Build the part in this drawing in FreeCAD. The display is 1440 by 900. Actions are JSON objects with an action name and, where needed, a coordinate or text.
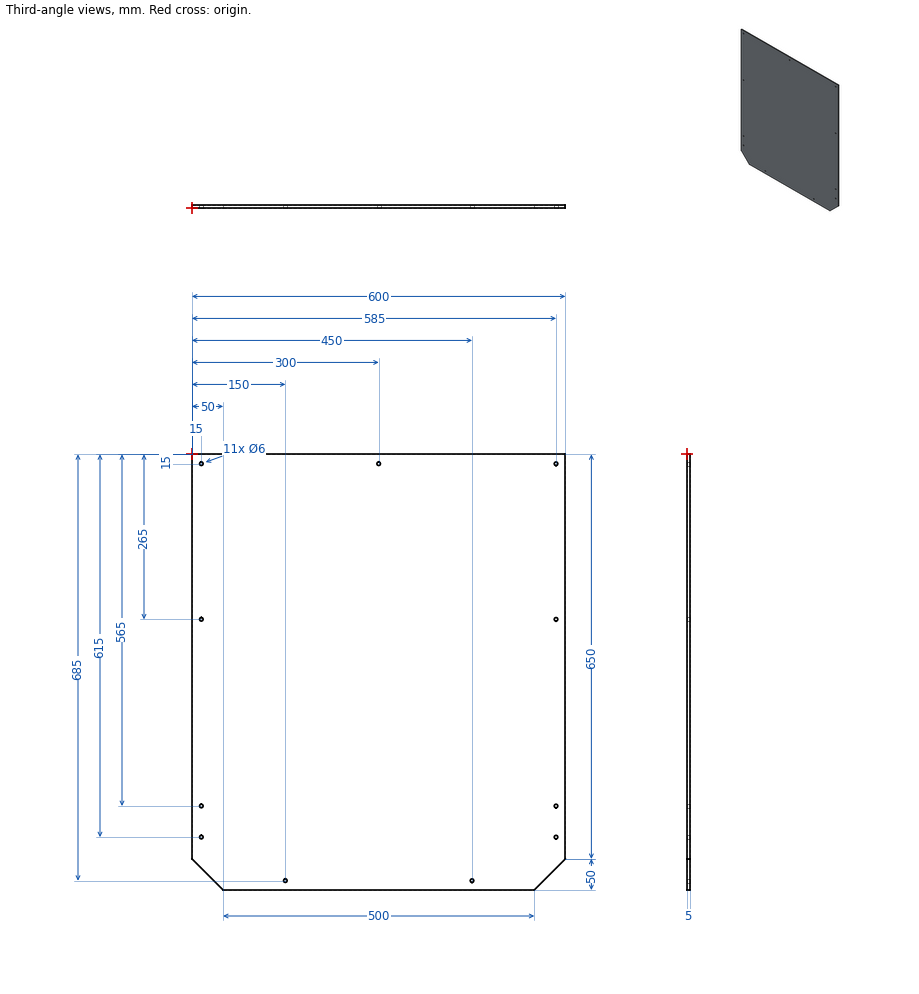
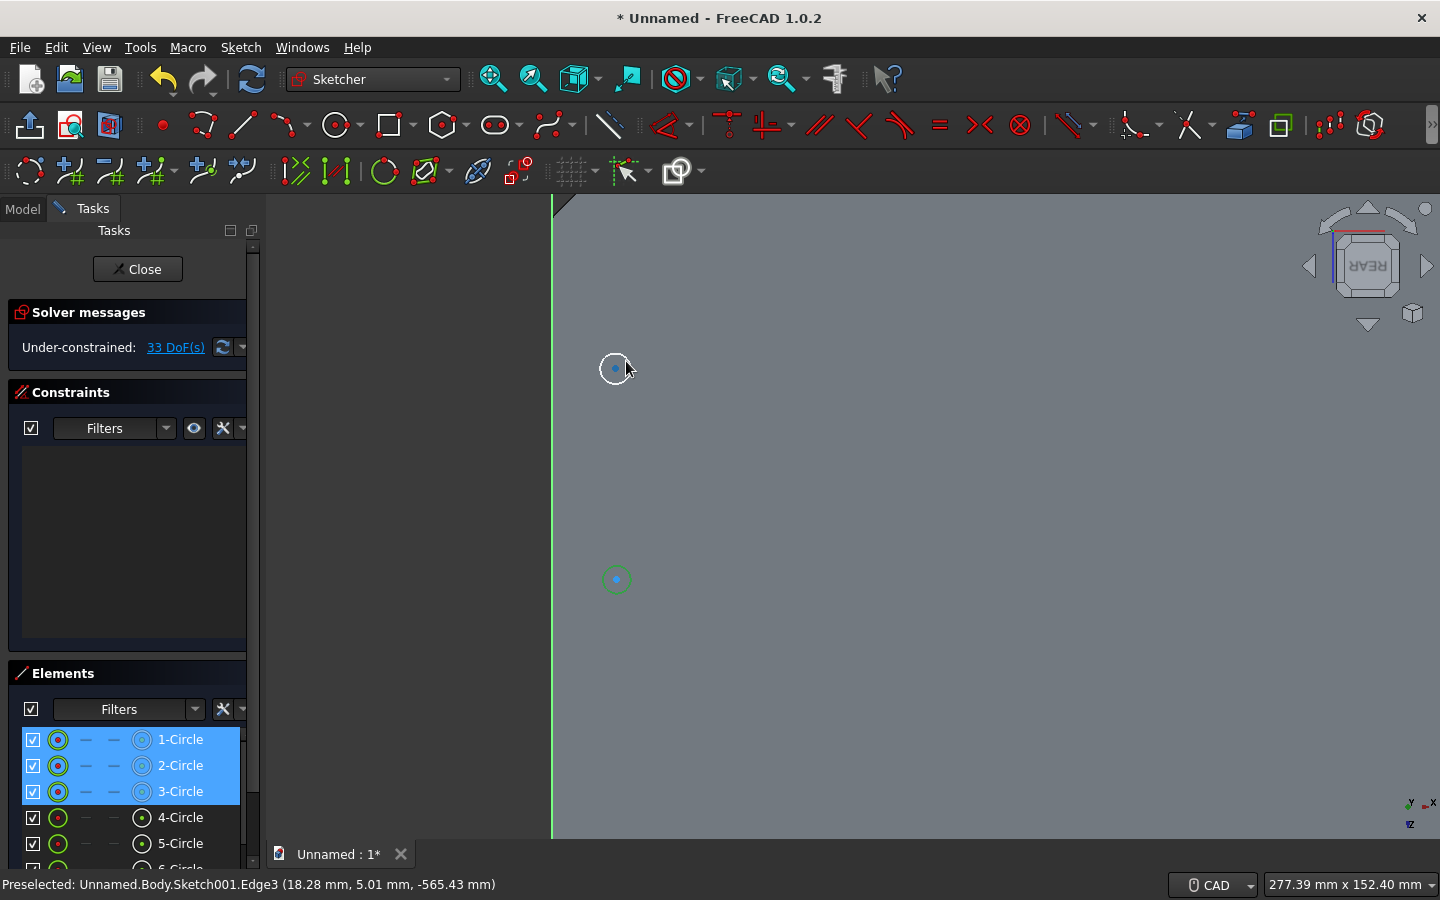
{"action": "left_click", "coordinate": [626, 358]}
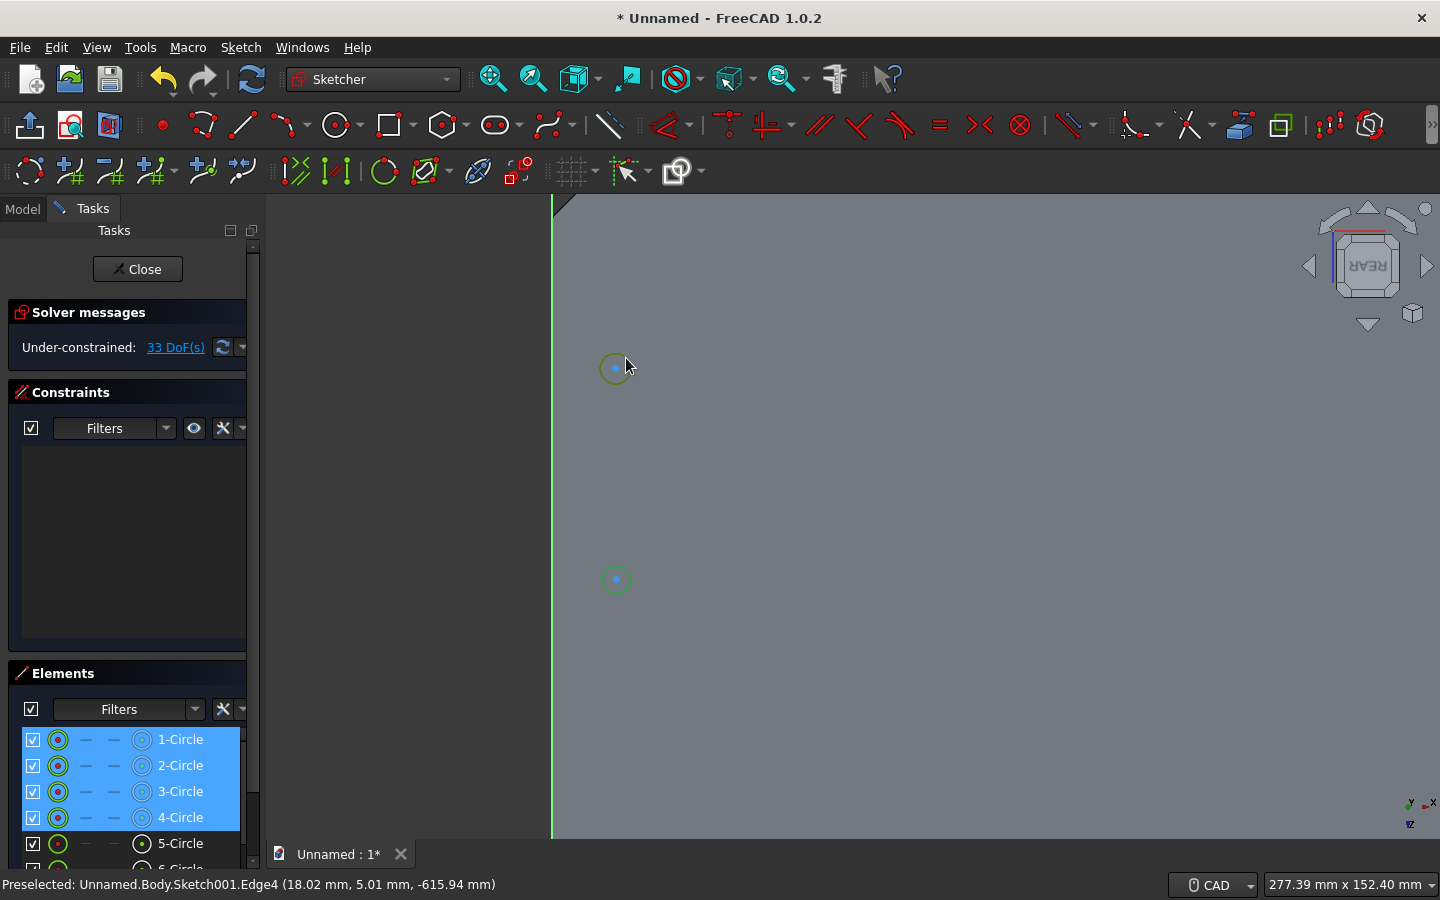
{"action": "scroll", "coordinate": [626, 361], "scroll_direction": "down", "scroll_amount": 10}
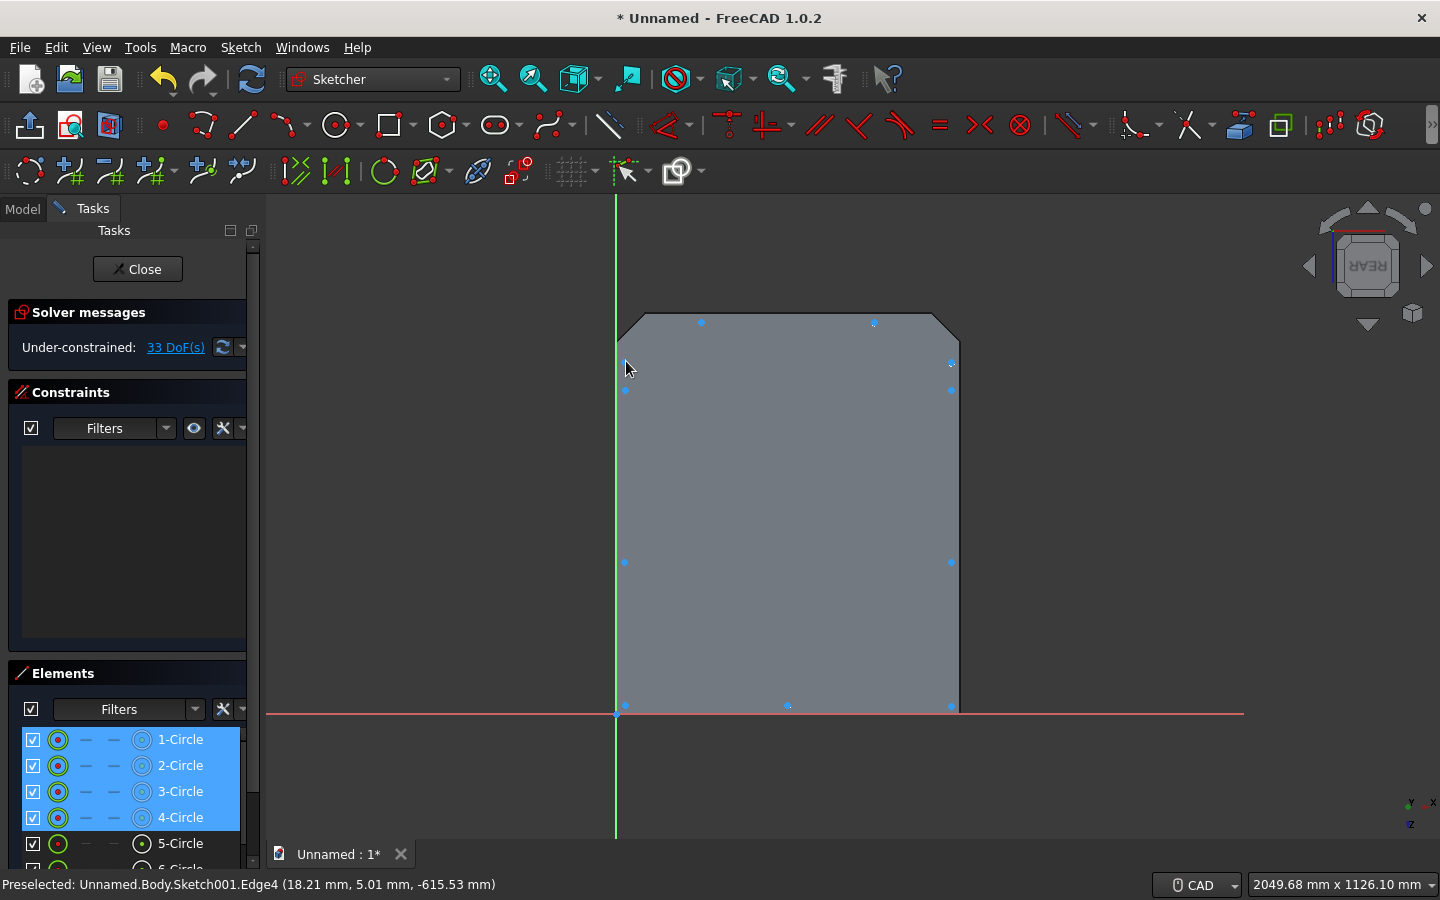
{"action": "scroll", "coordinate": [704, 321], "scroll_direction": "up", "scroll_amount": 9}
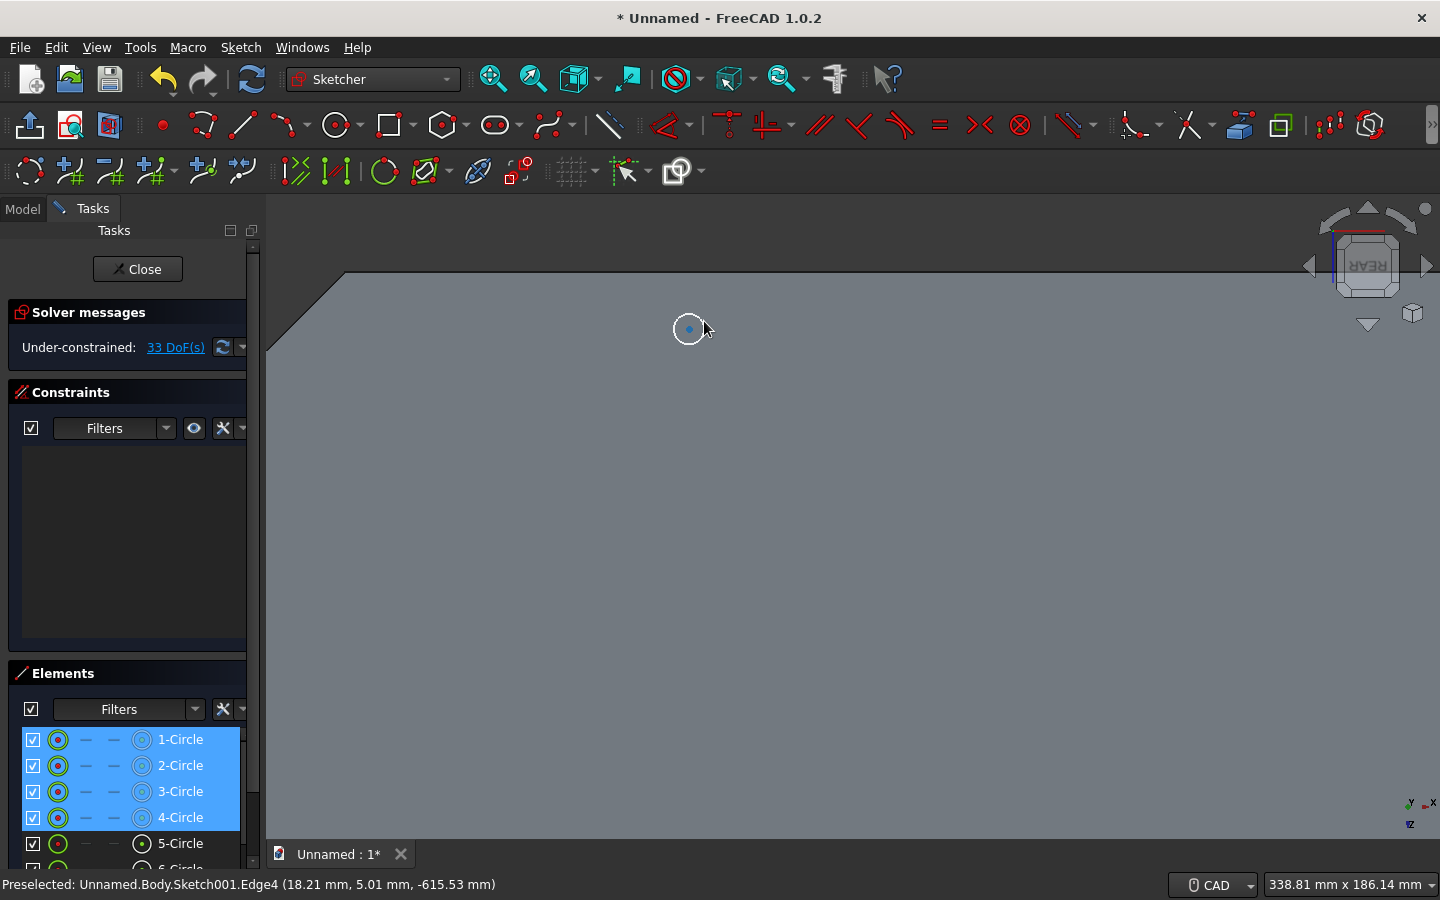
{"action": "left_click", "coordinate": [700, 318]}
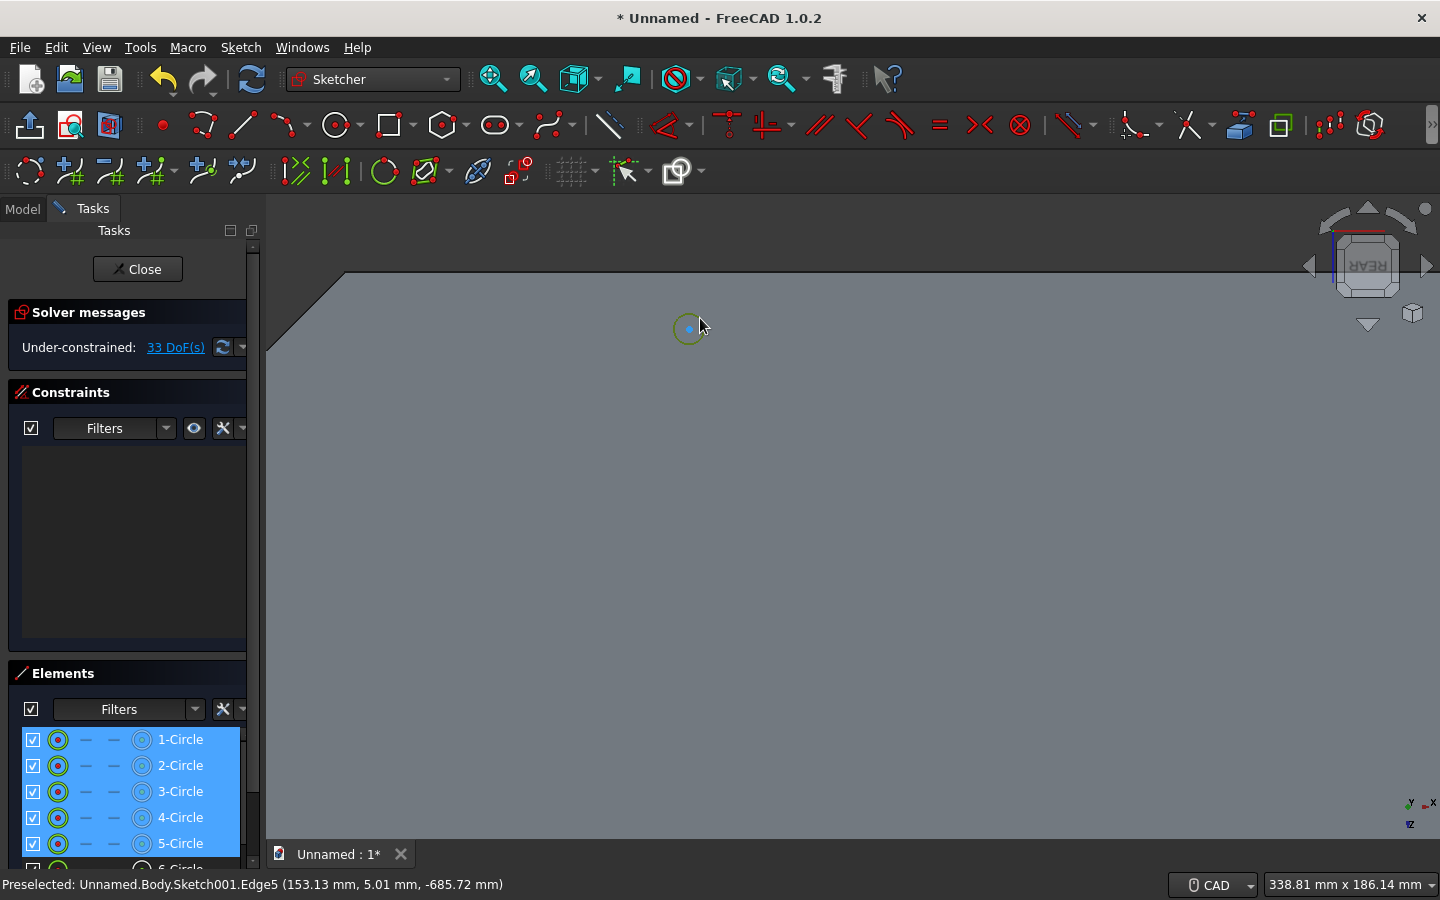
{"action": "scroll", "coordinate": [704, 321], "scroll_direction": "down", "scroll_amount": 9}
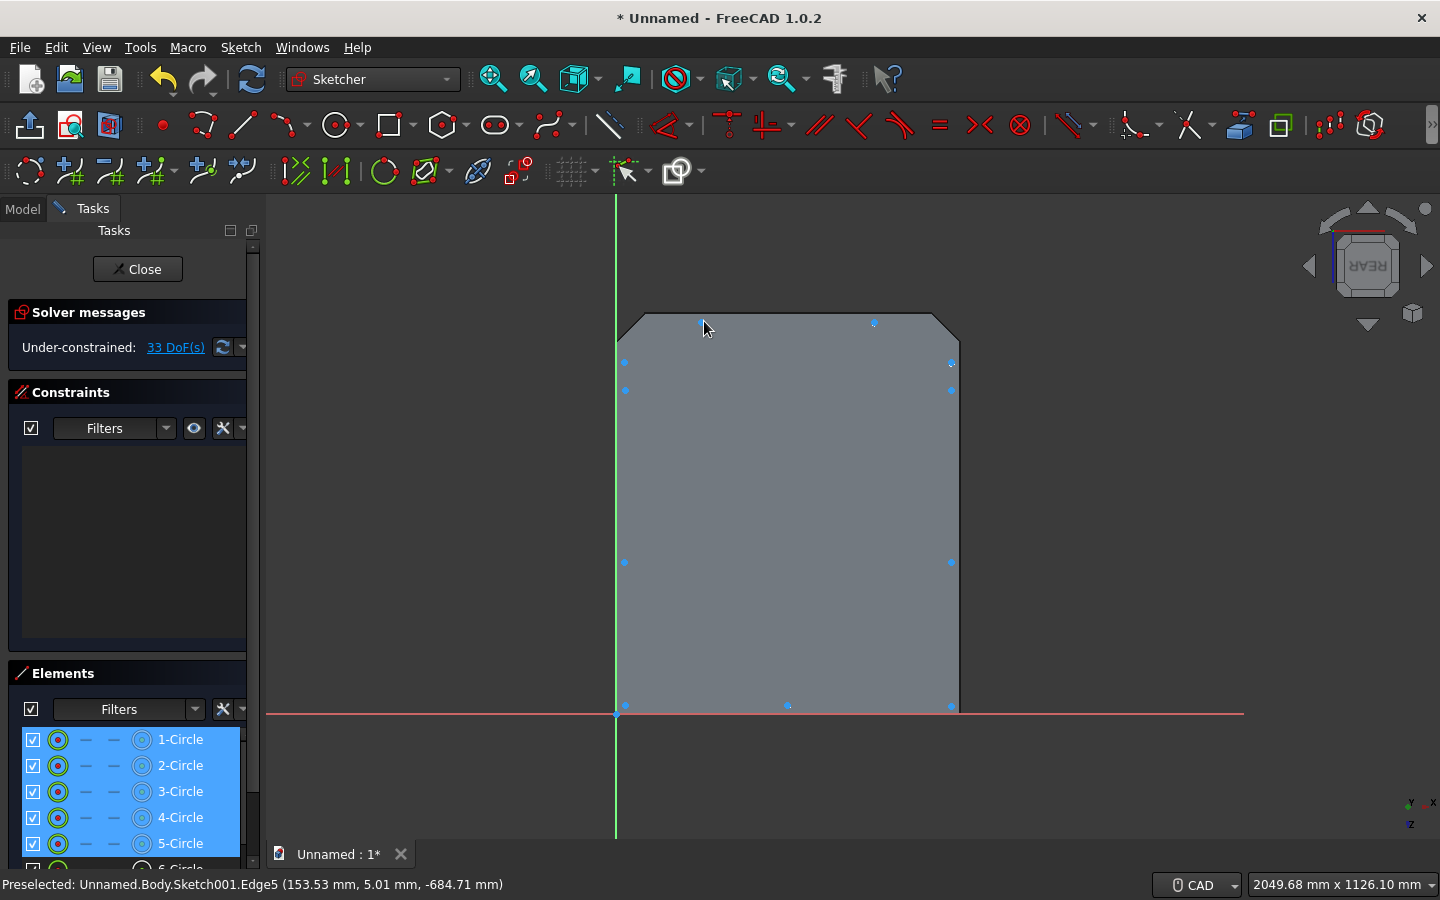
{"action": "scroll", "coordinate": [953, 704], "scroll_direction": "up", "scroll_amount": 10}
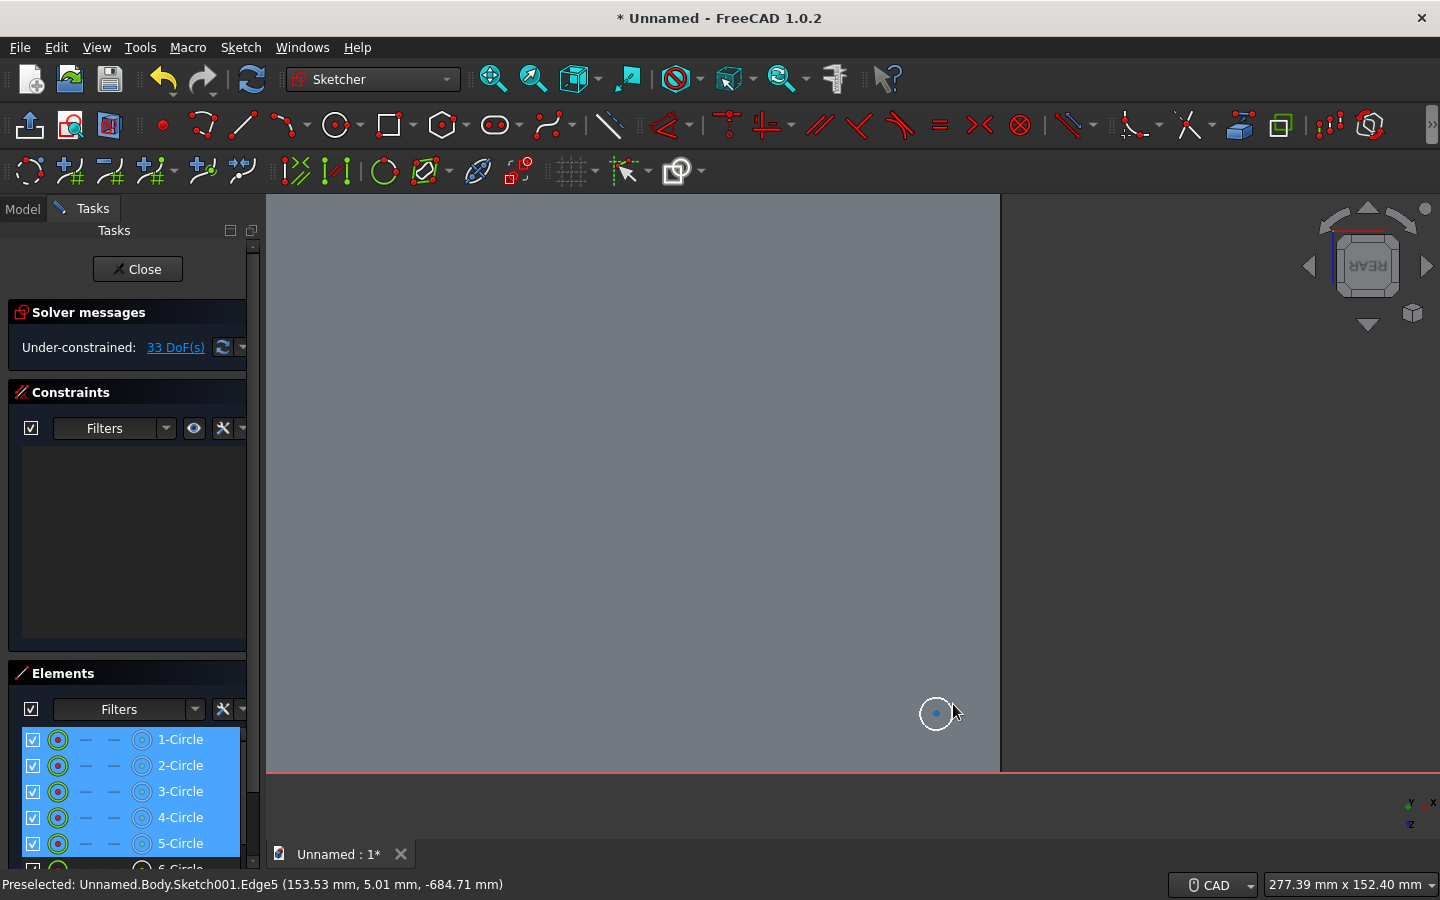
{"action": "left_click", "coordinate": [948, 702]}